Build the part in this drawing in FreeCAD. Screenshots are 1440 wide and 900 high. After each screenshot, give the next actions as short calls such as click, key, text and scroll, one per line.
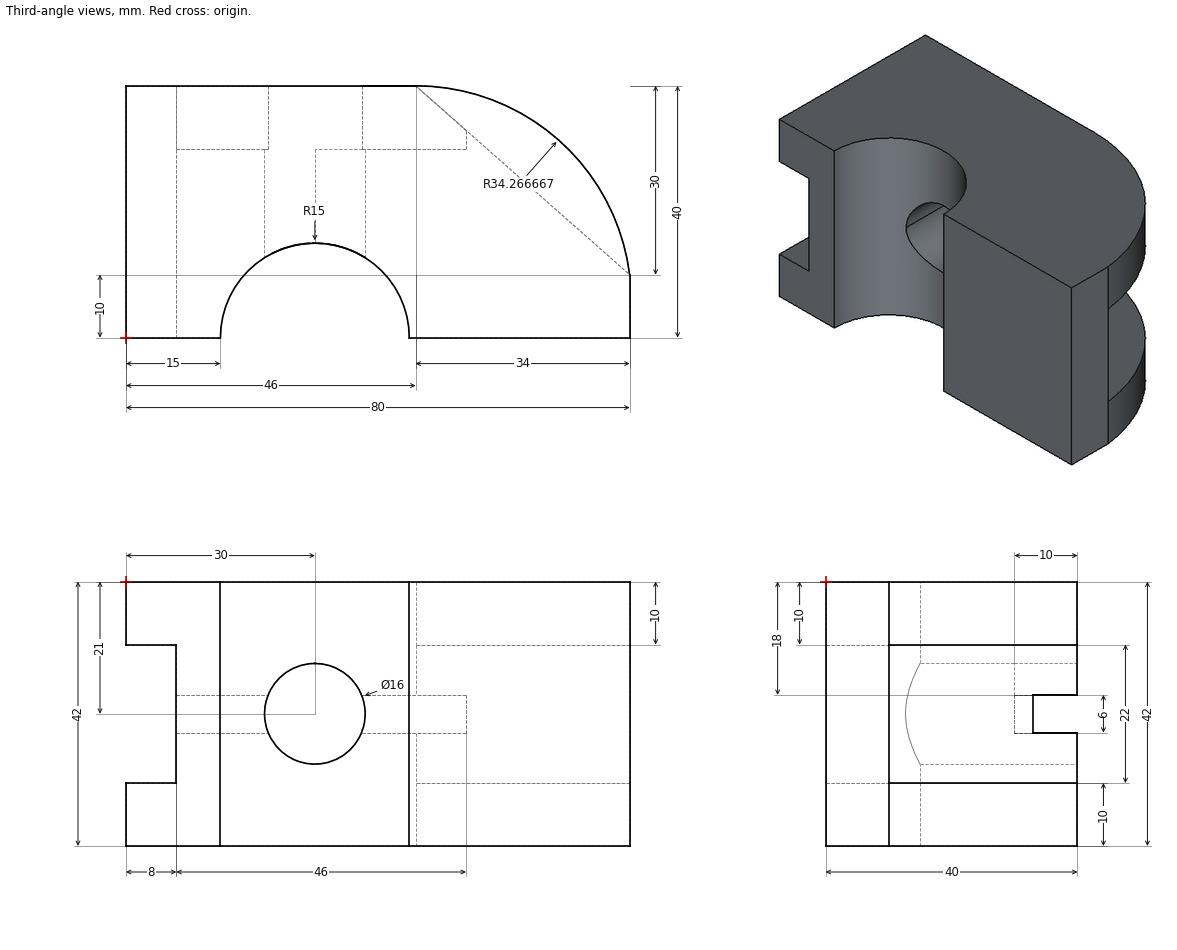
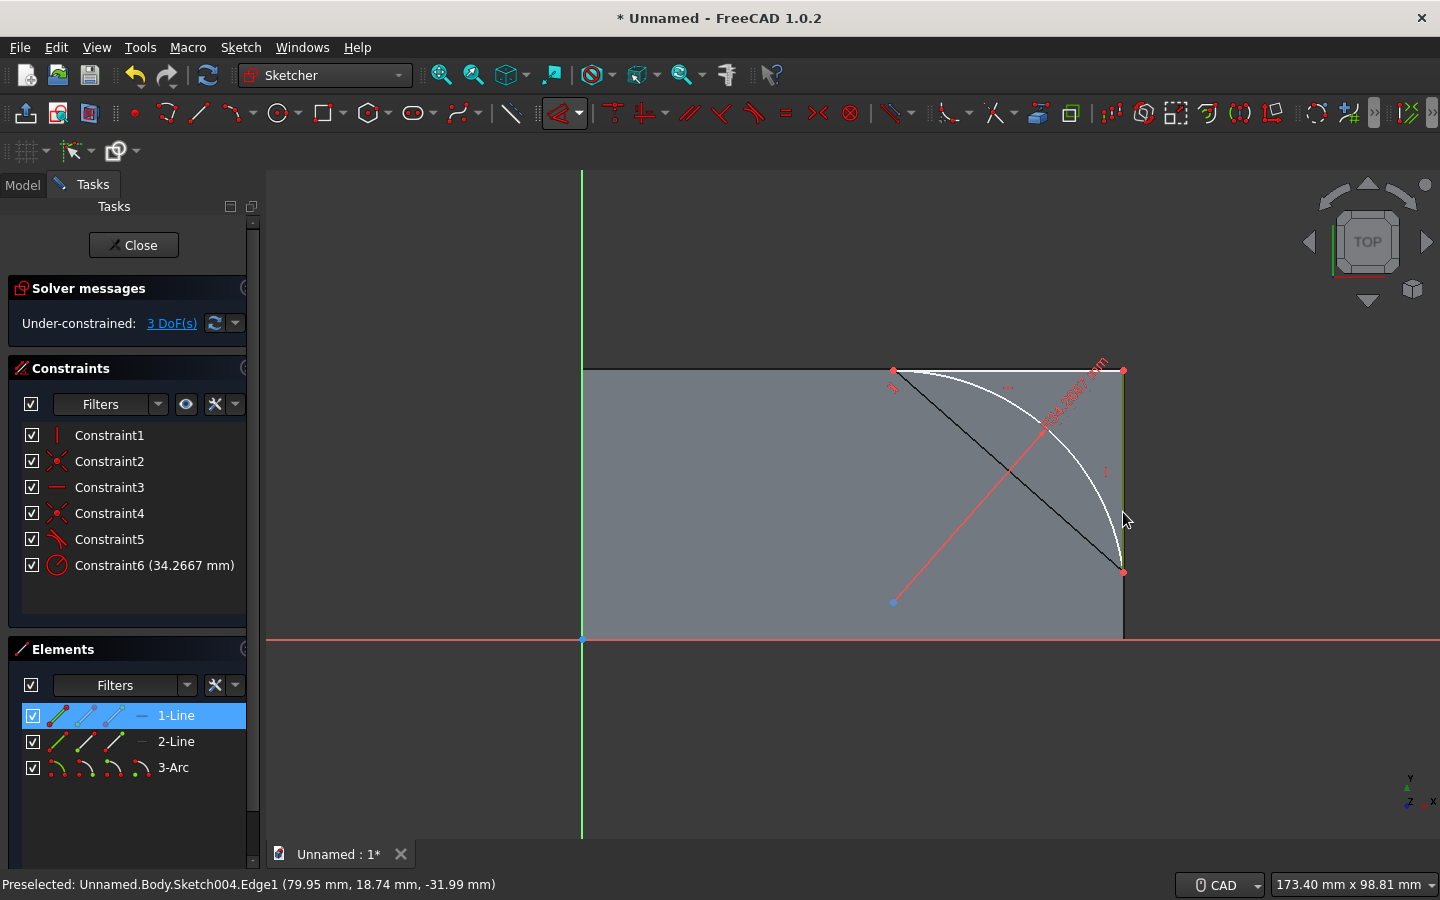
click(582, 114)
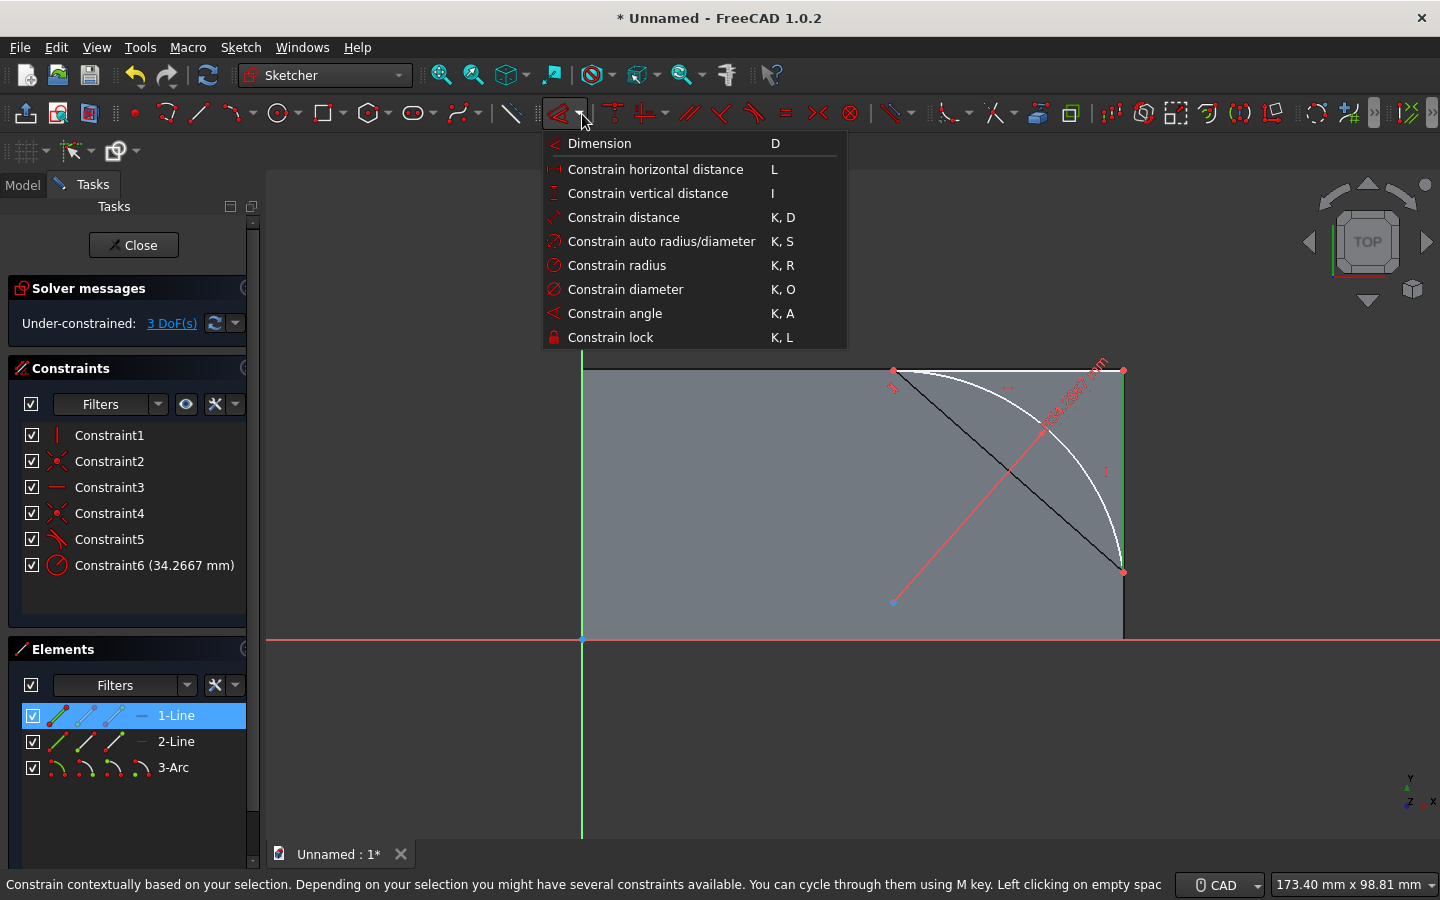
click(695, 193)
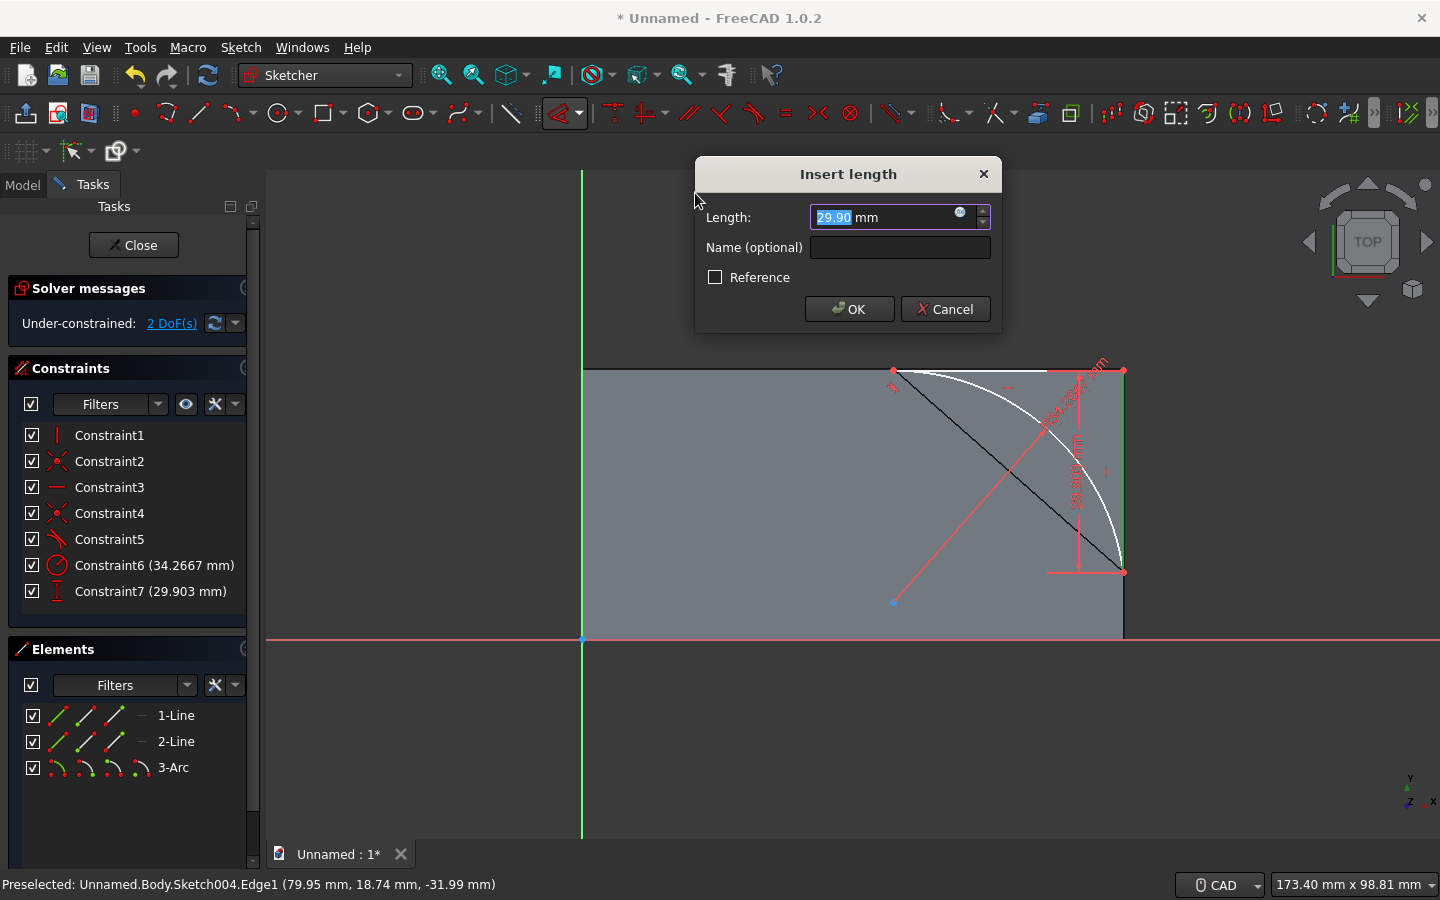
text(30)
key(Return)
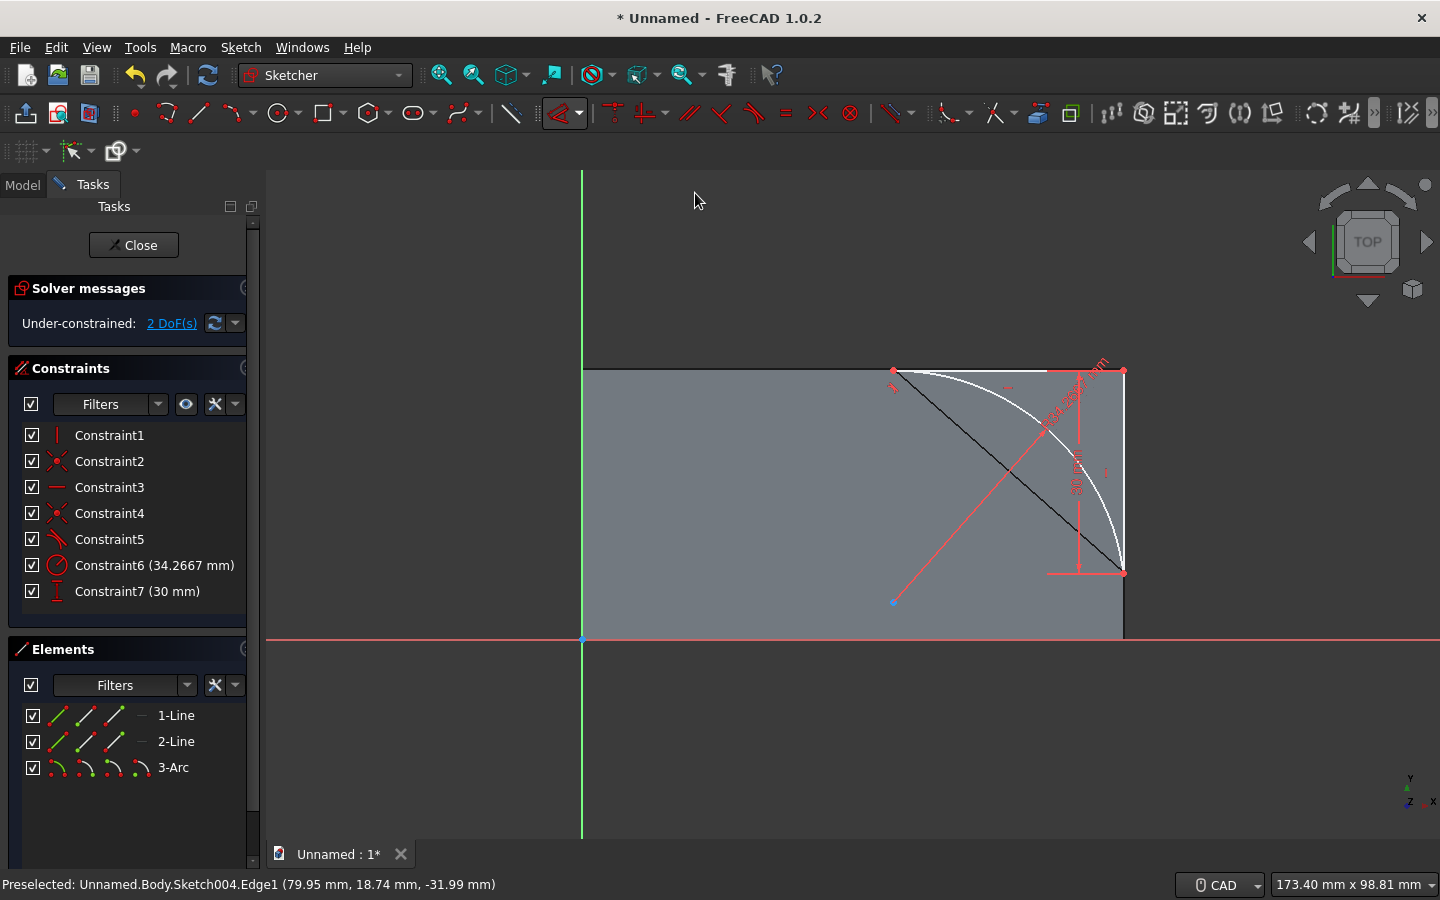
click(1124, 574)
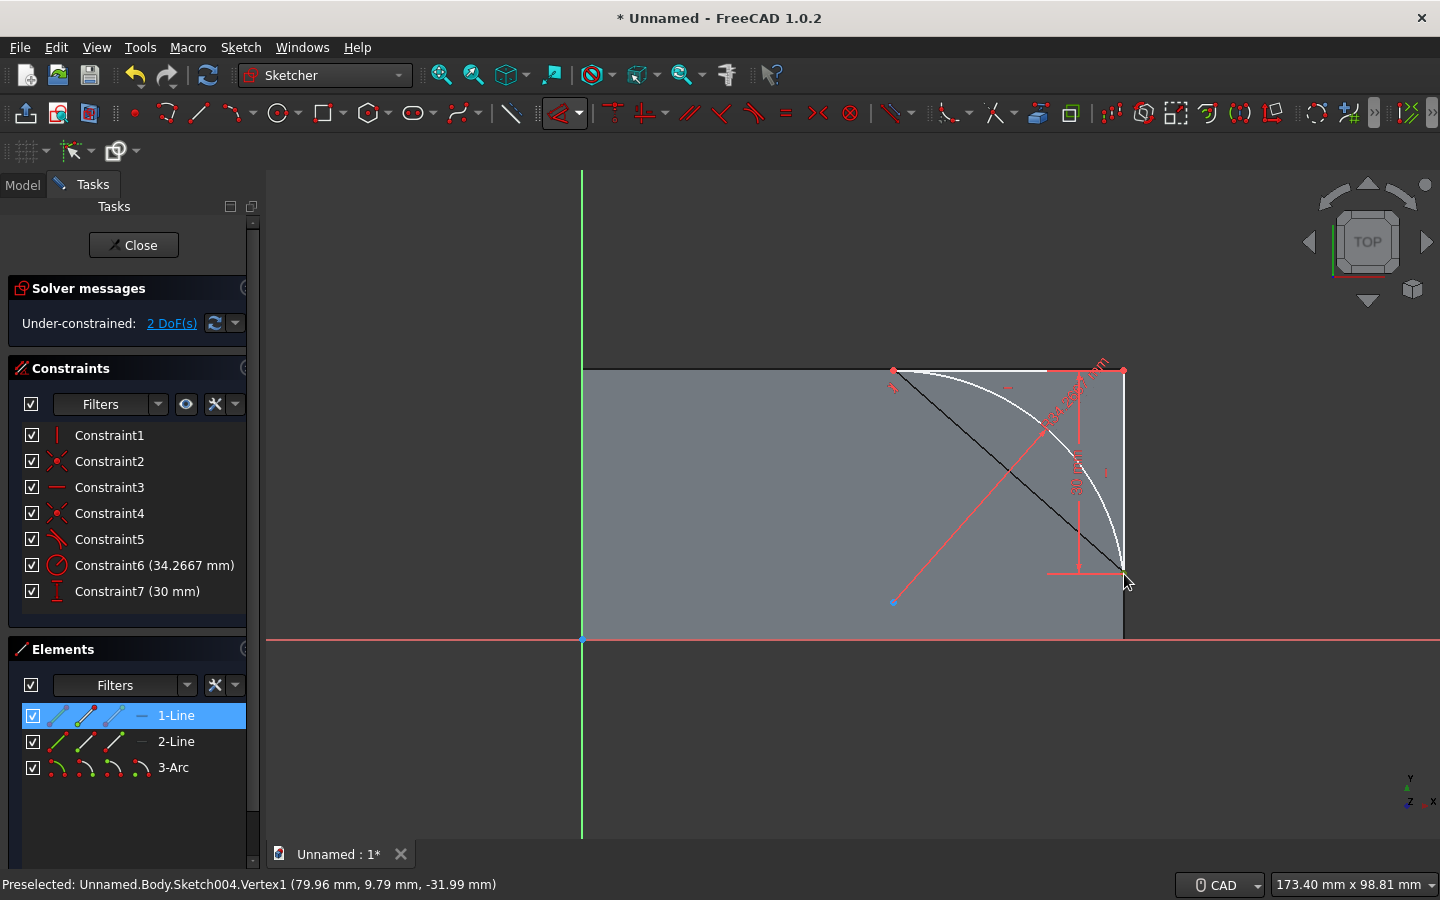
click(582, 114)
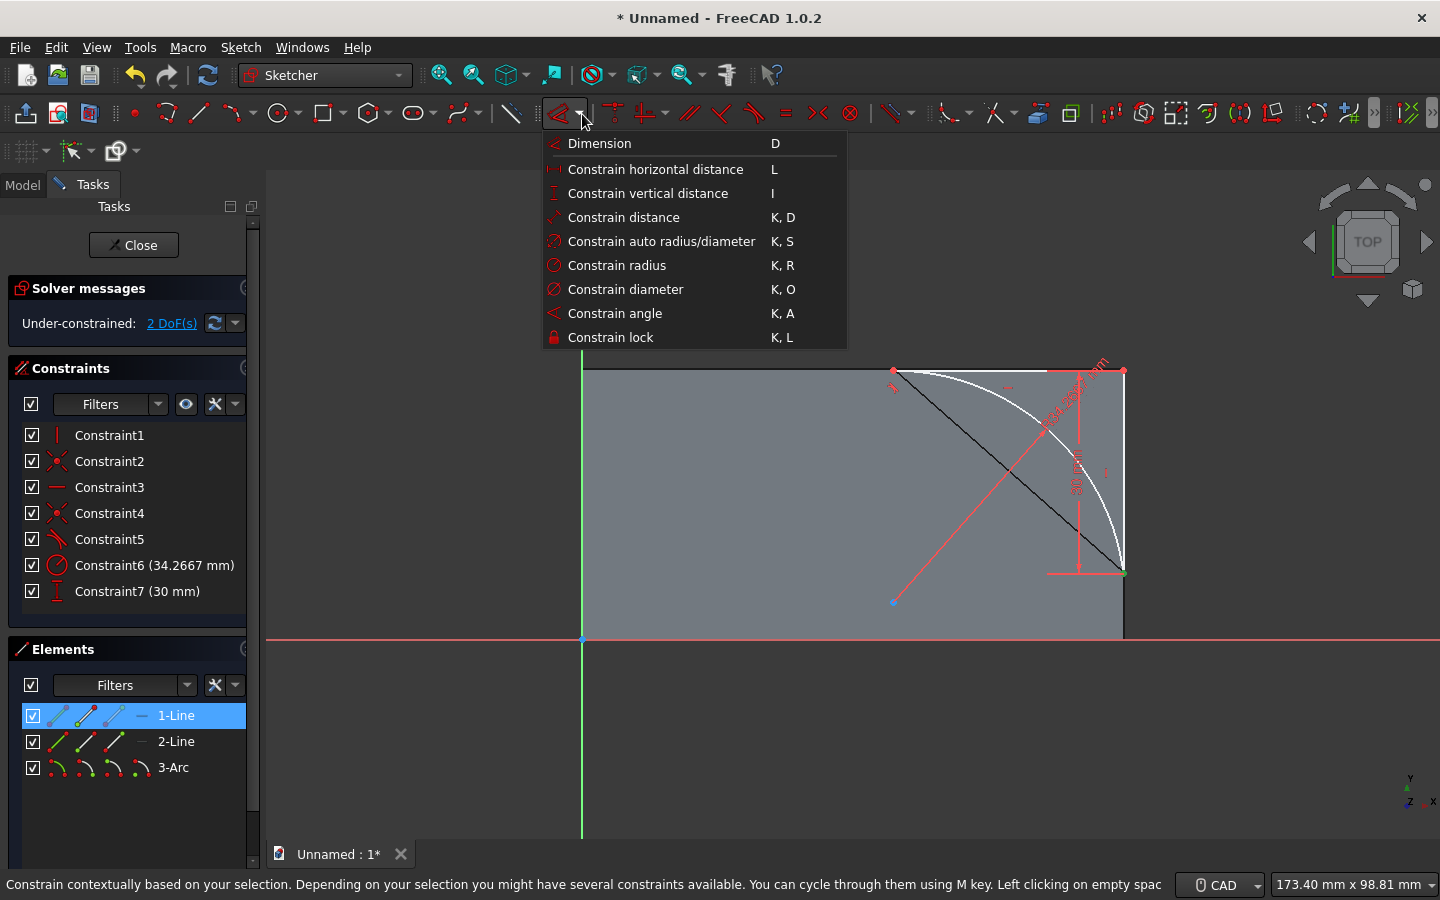
click(695, 169)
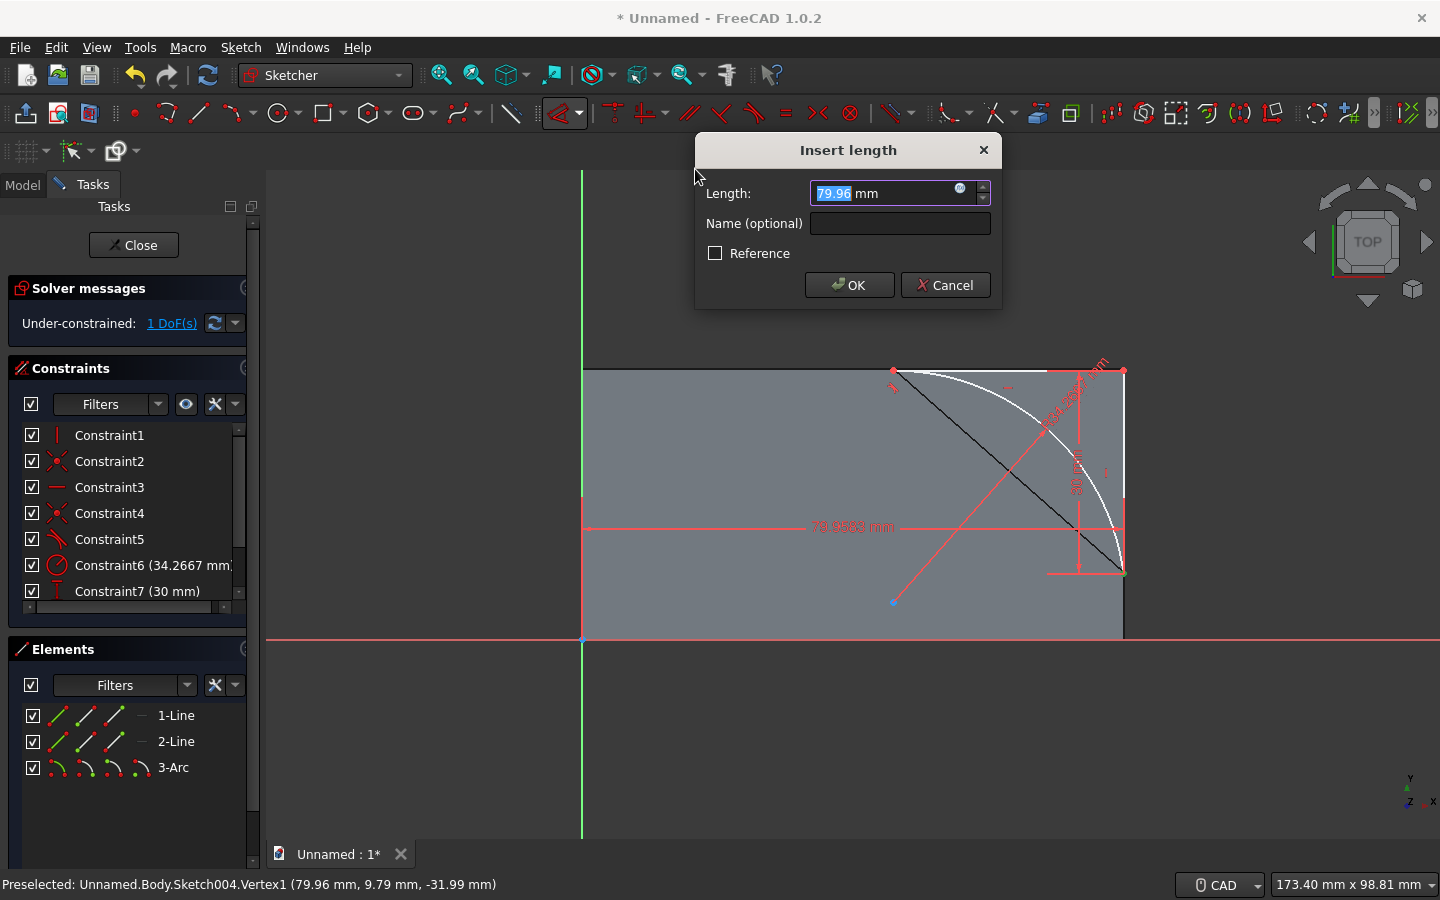
text(80)
key(Return)